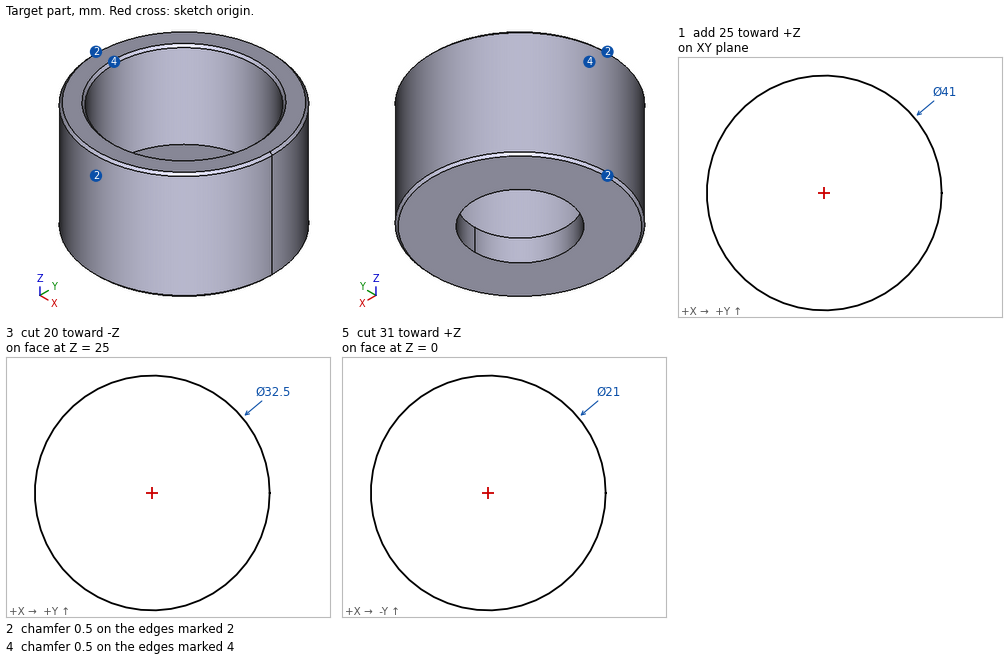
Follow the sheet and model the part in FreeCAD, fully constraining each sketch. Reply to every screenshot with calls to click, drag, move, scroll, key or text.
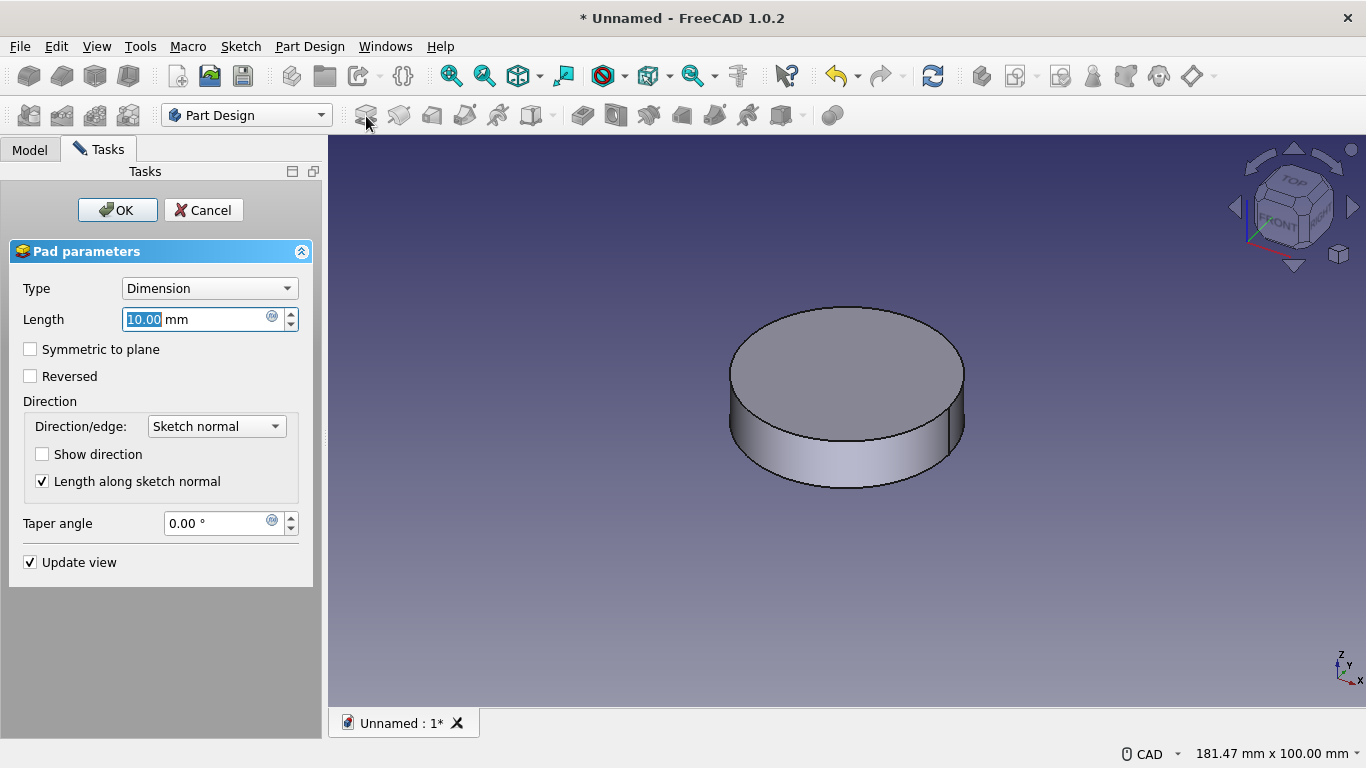
text(25)
key(Tab)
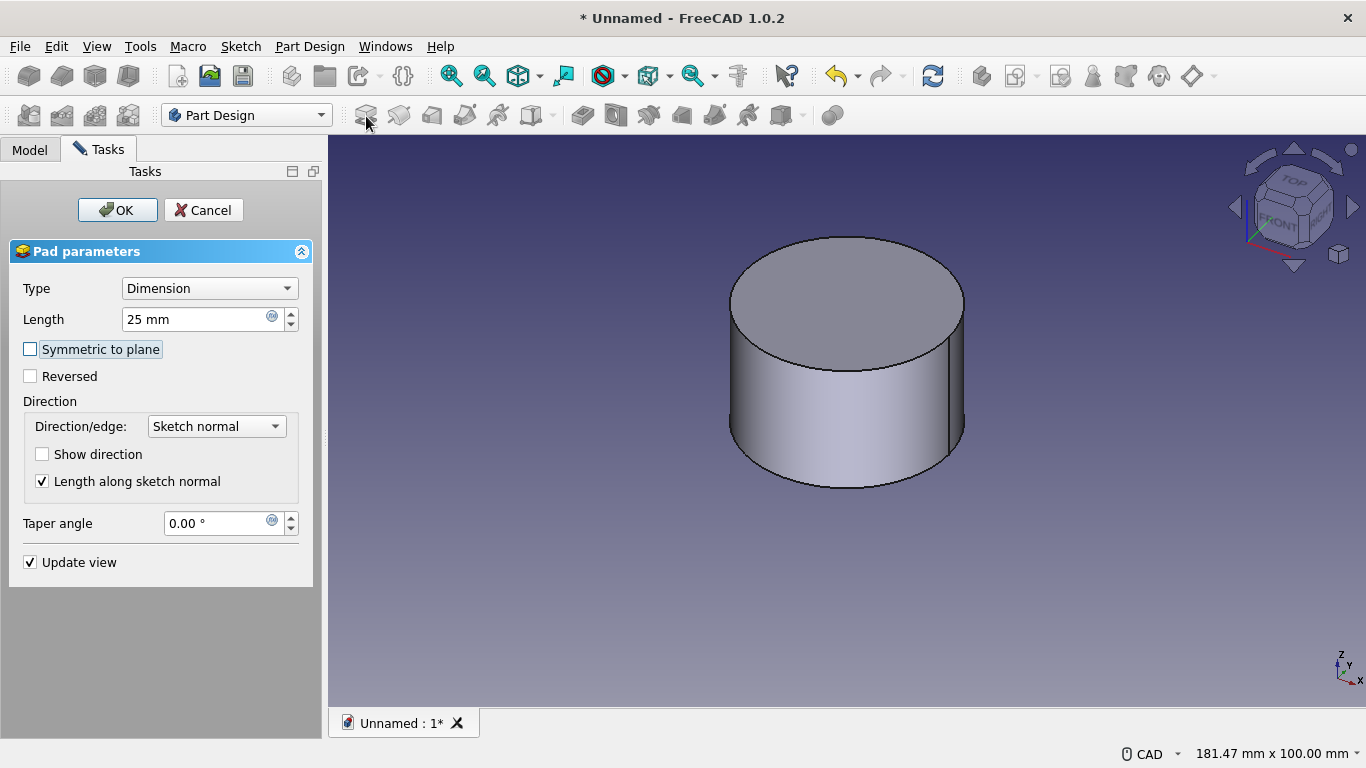
click(118, 210)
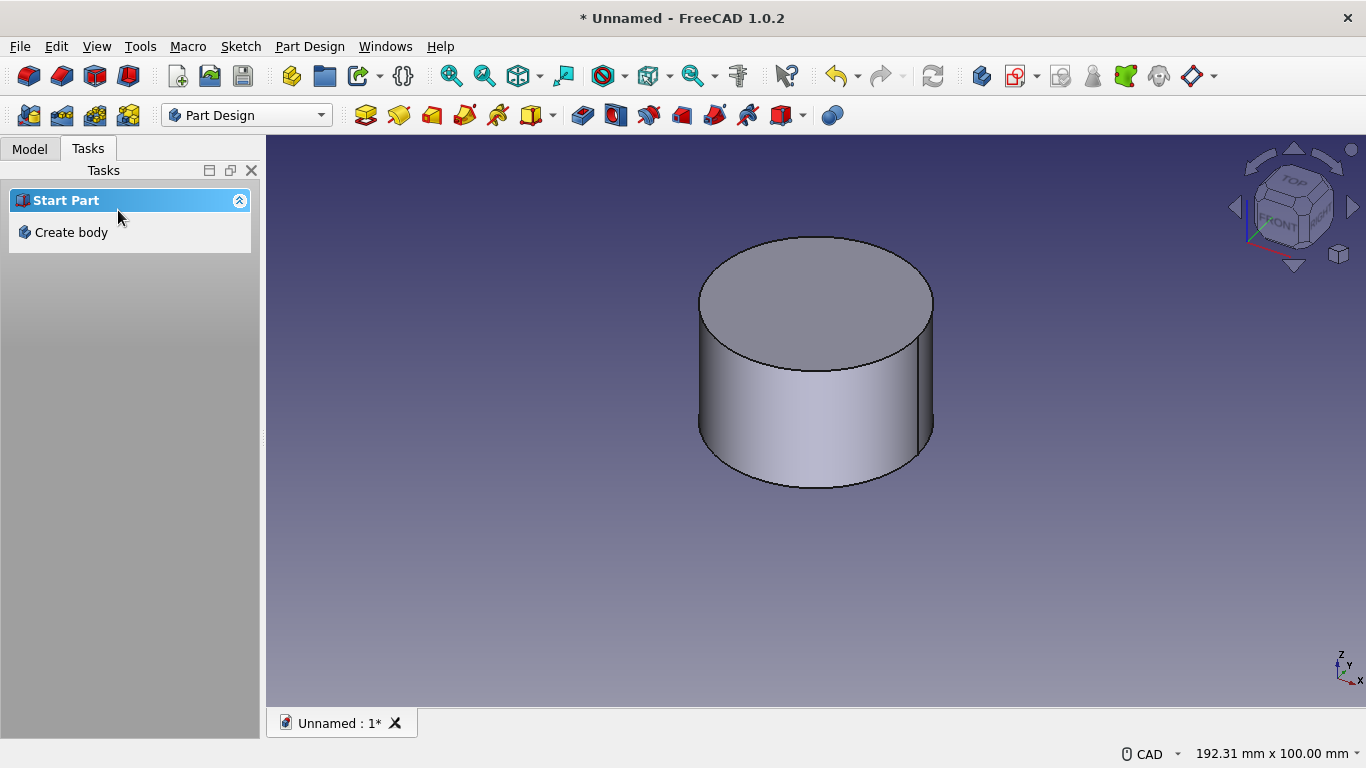
click(699, 310)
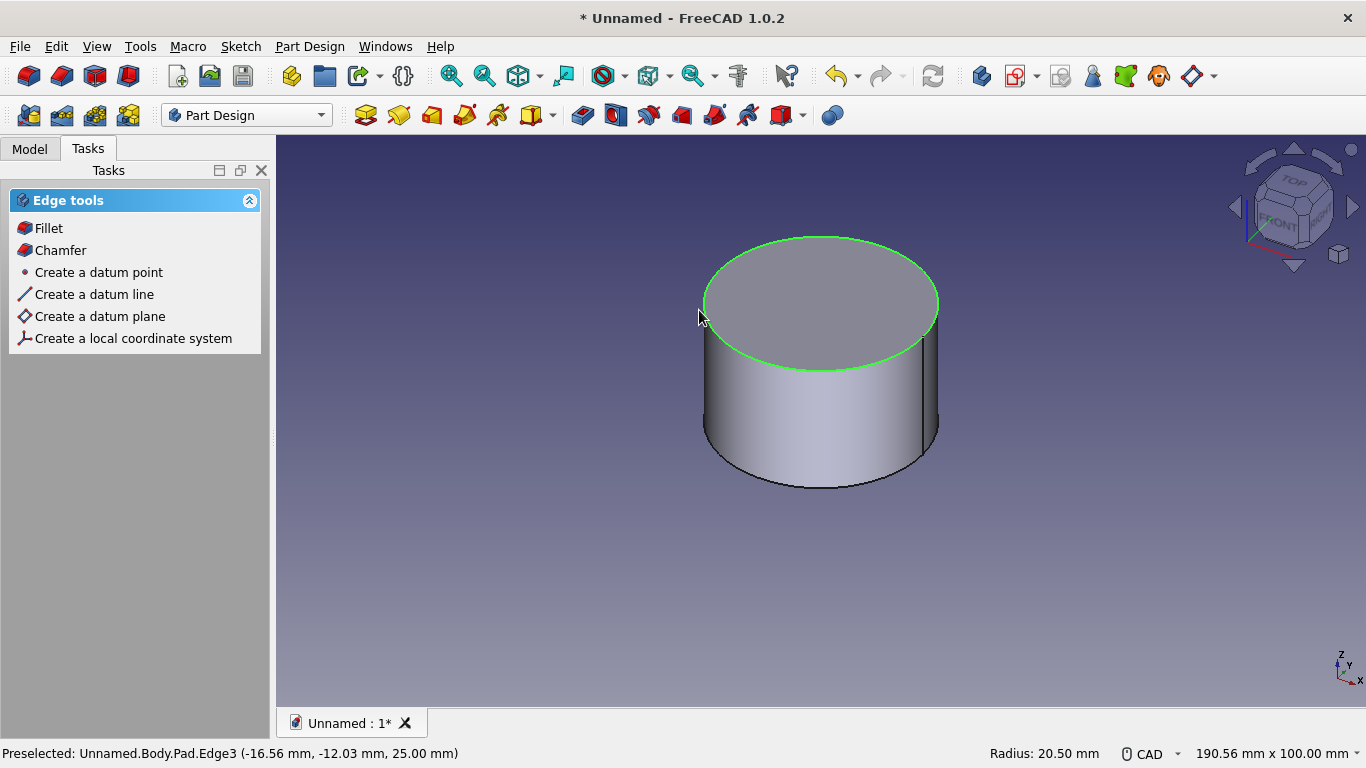
key(0)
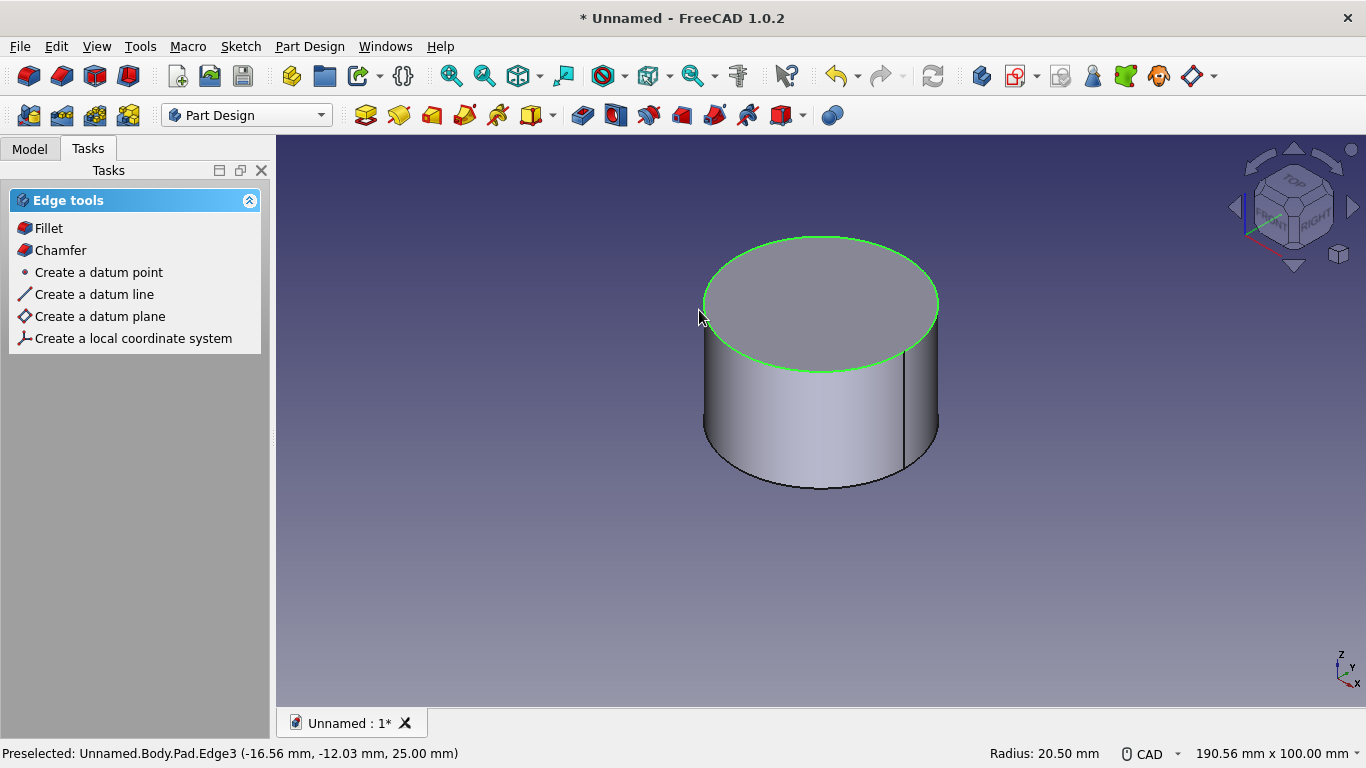
key(2)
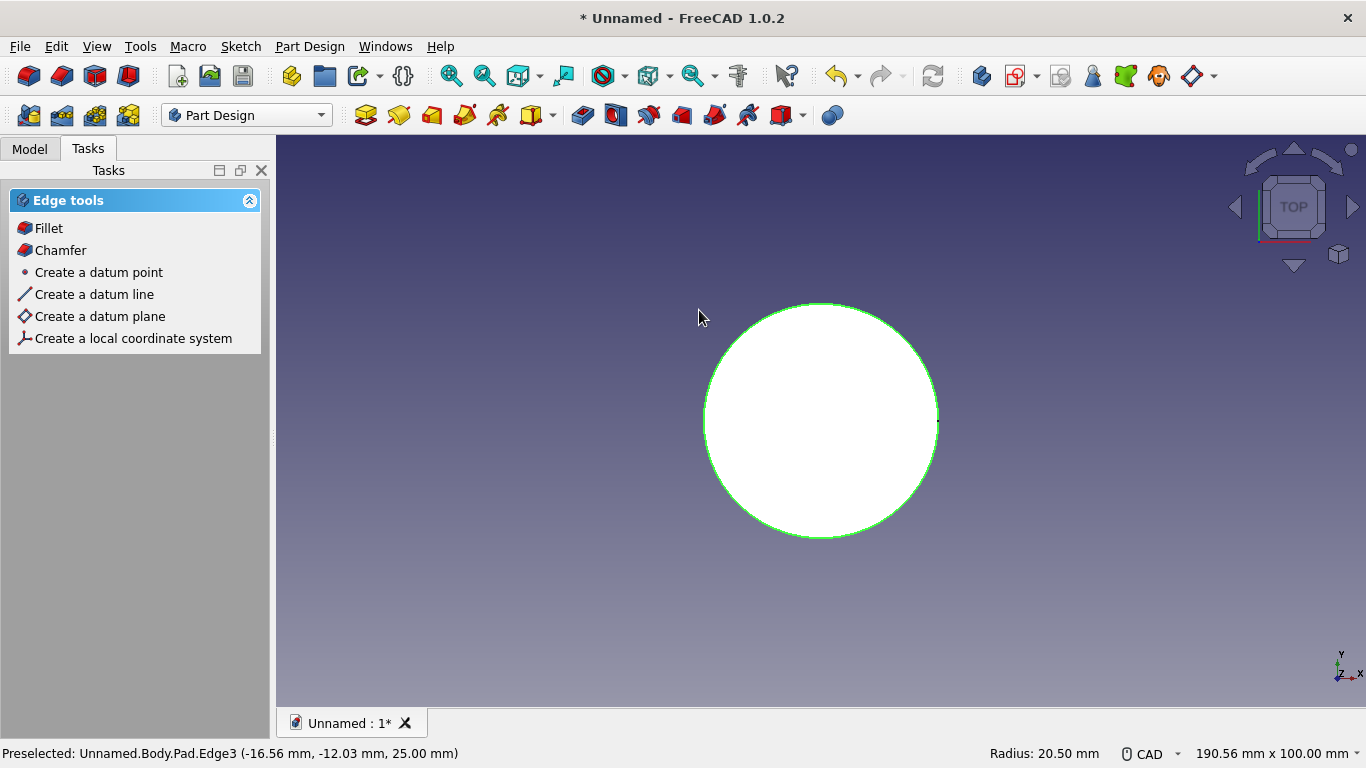
click(452, 76)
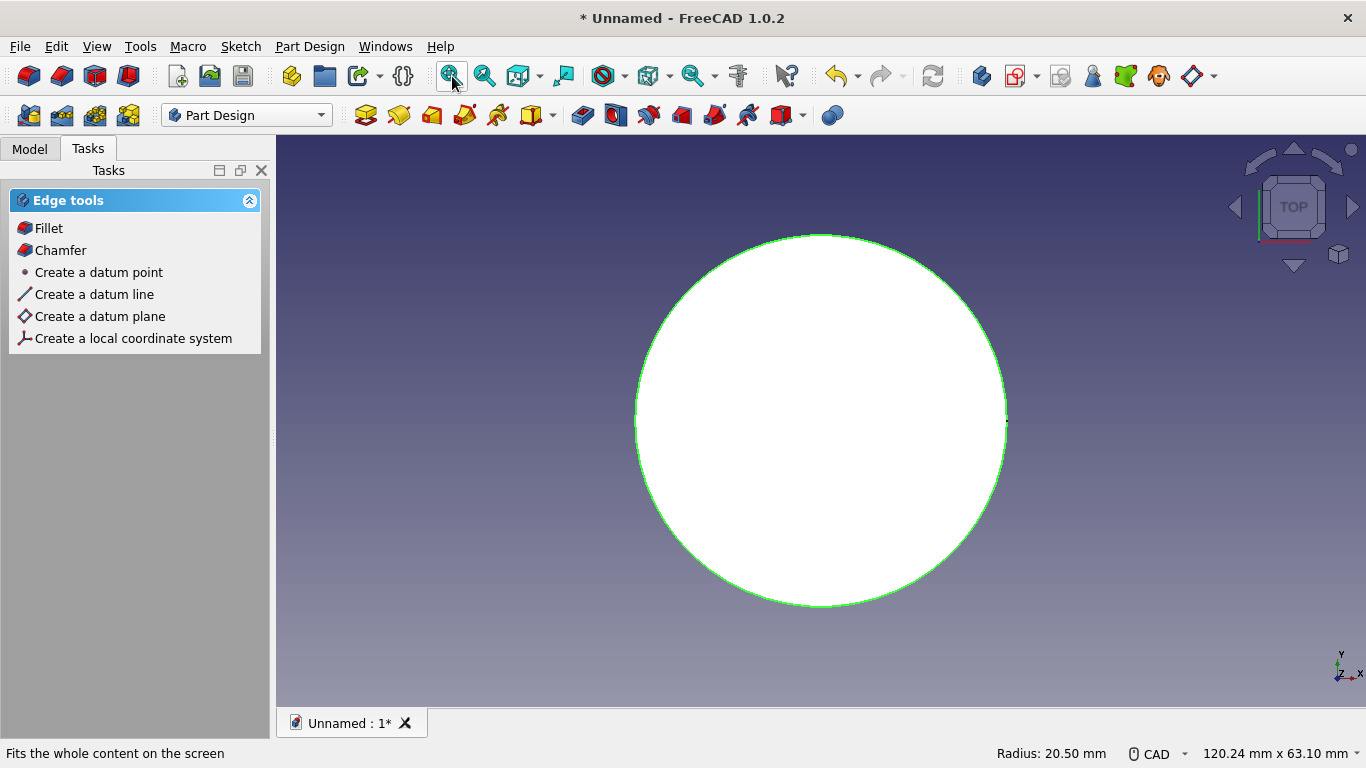
key(1)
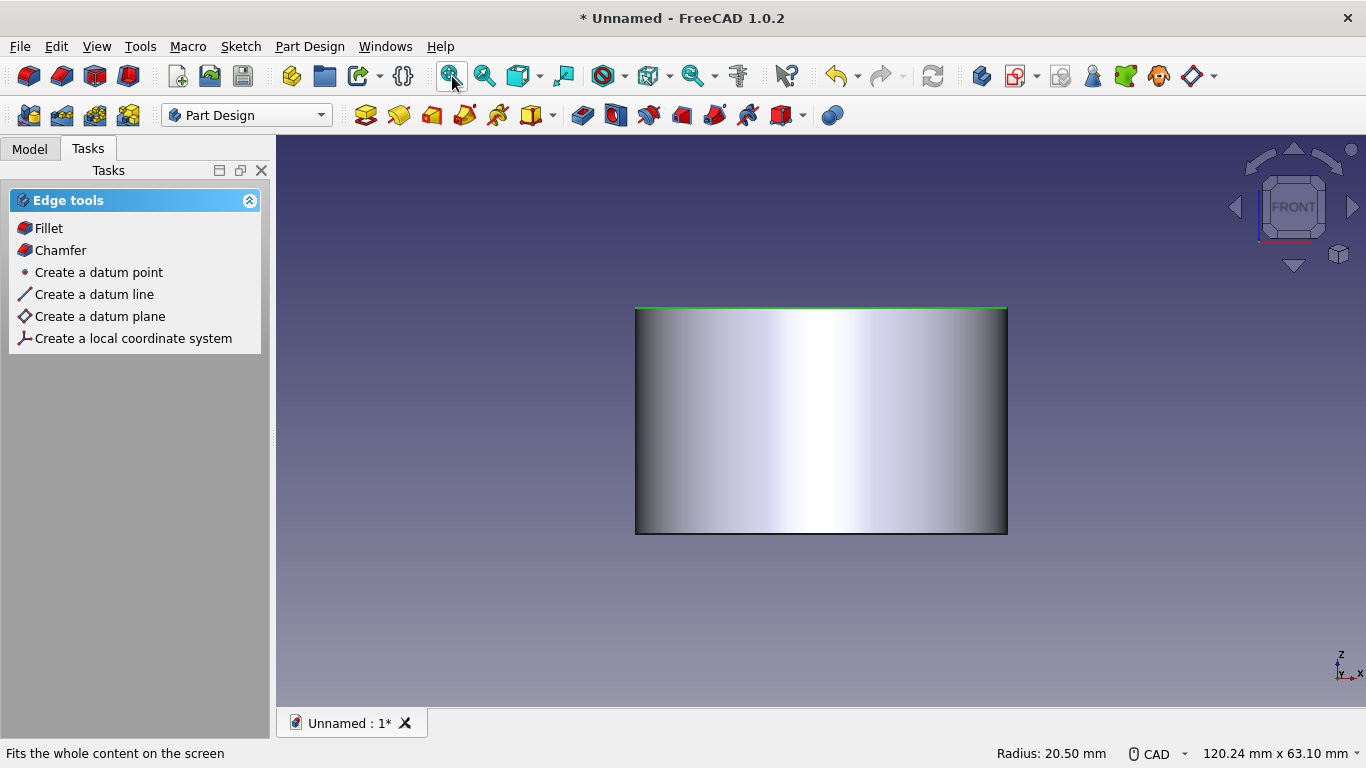
click(452, 76)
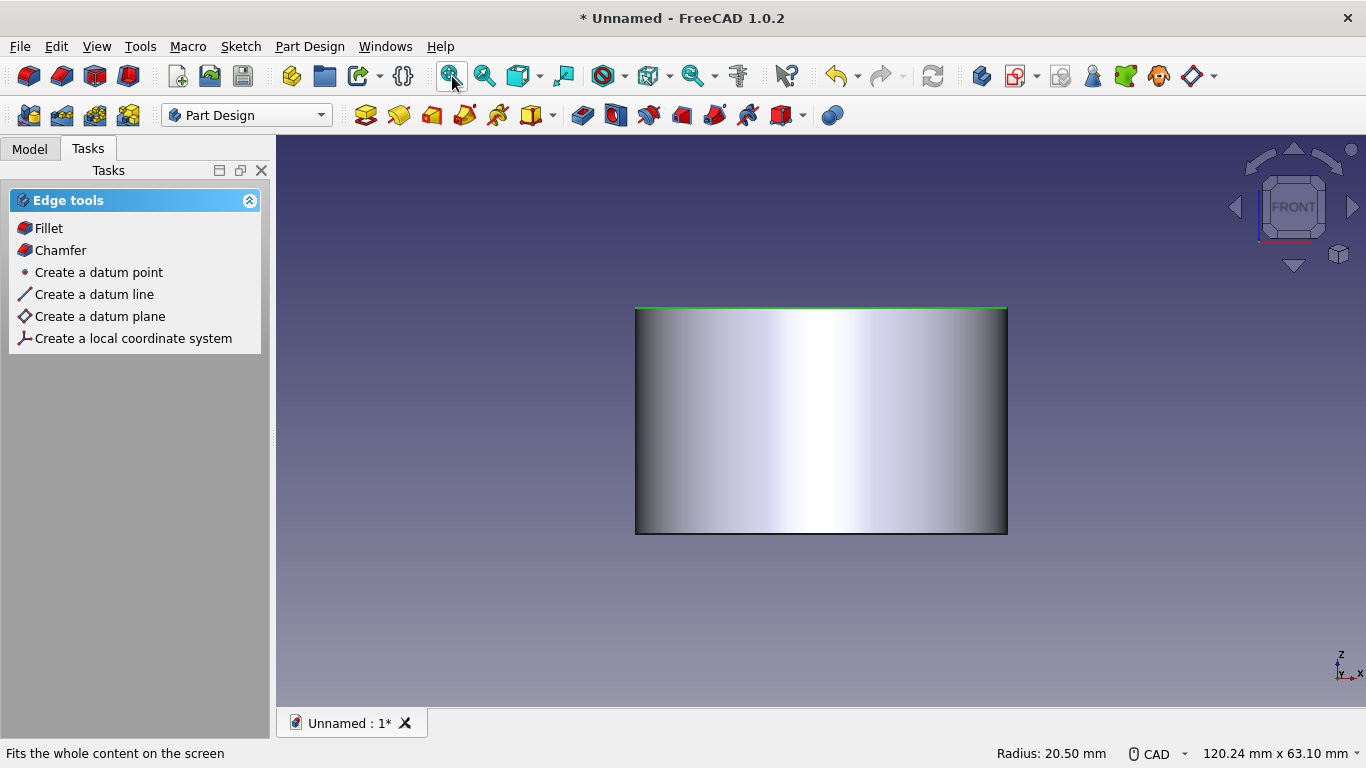
click(671, 533, ctrl)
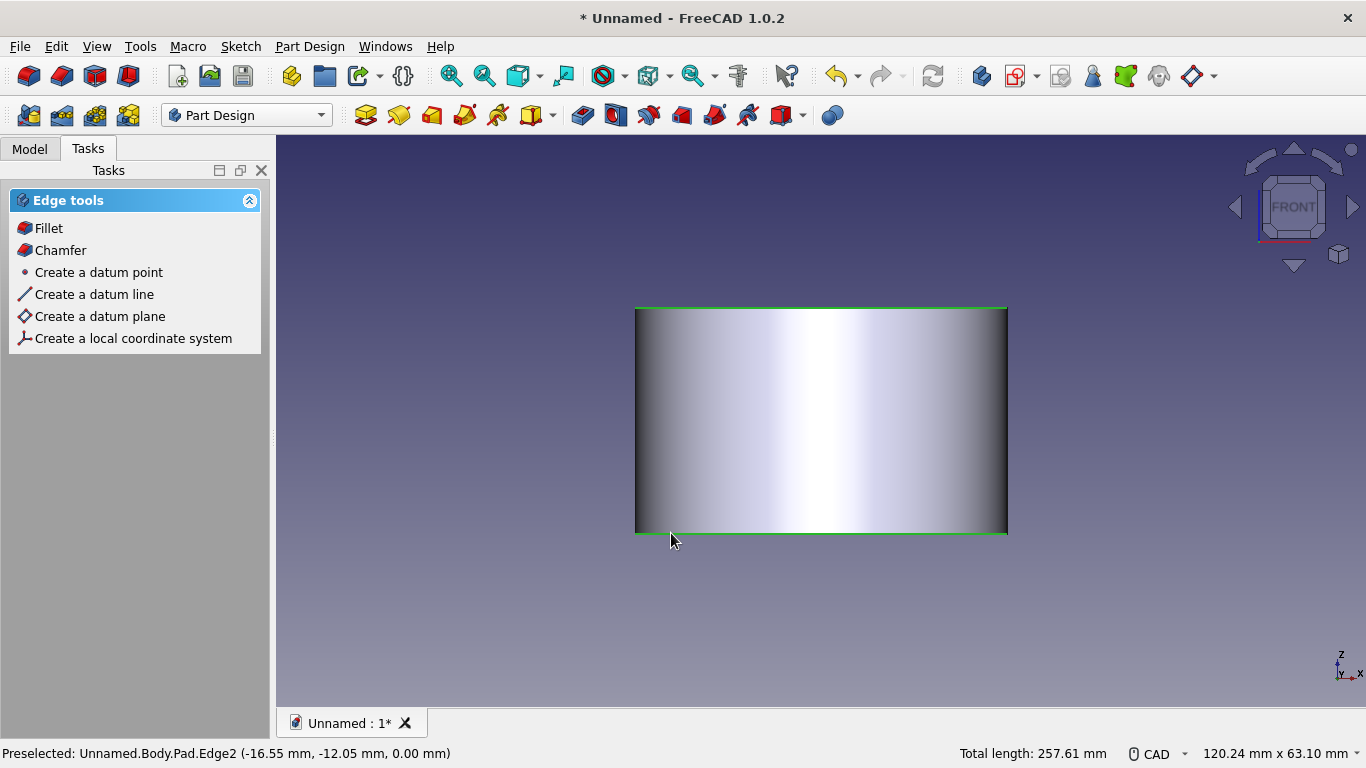
click(62, 76)